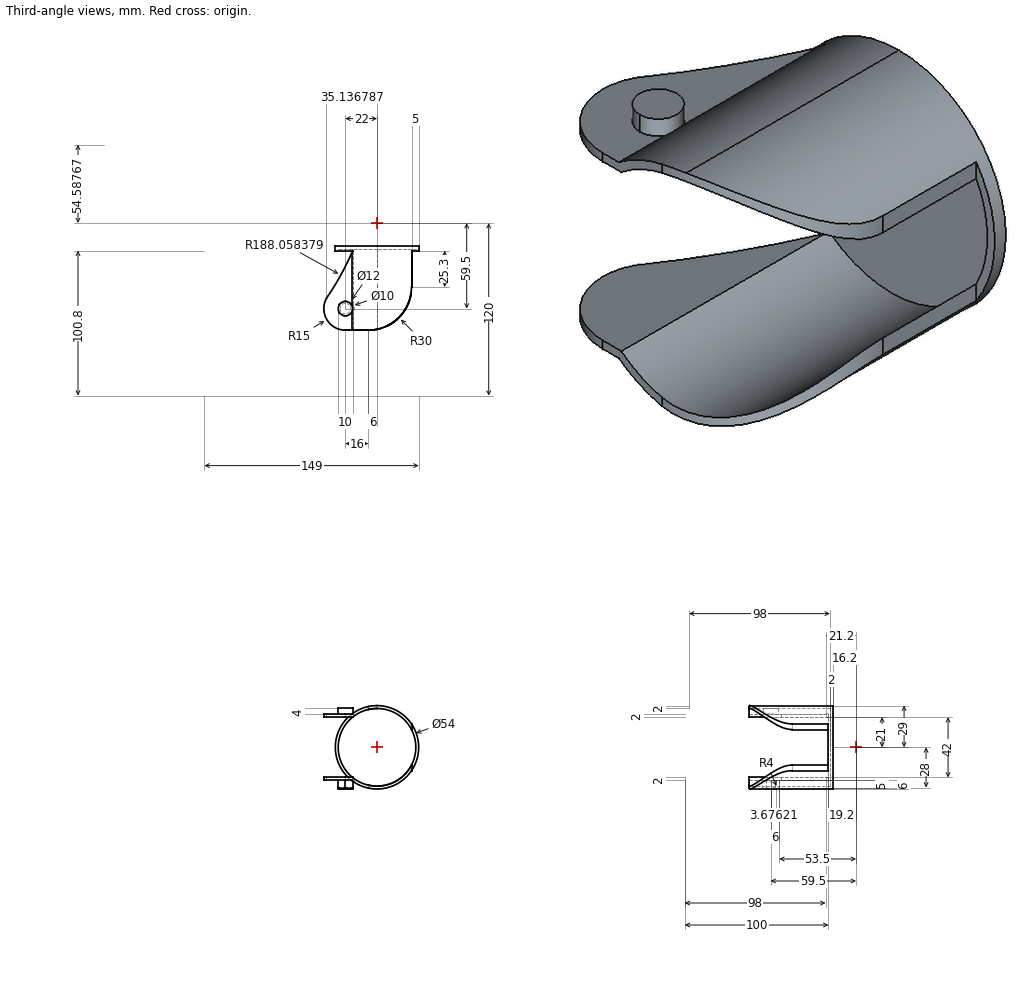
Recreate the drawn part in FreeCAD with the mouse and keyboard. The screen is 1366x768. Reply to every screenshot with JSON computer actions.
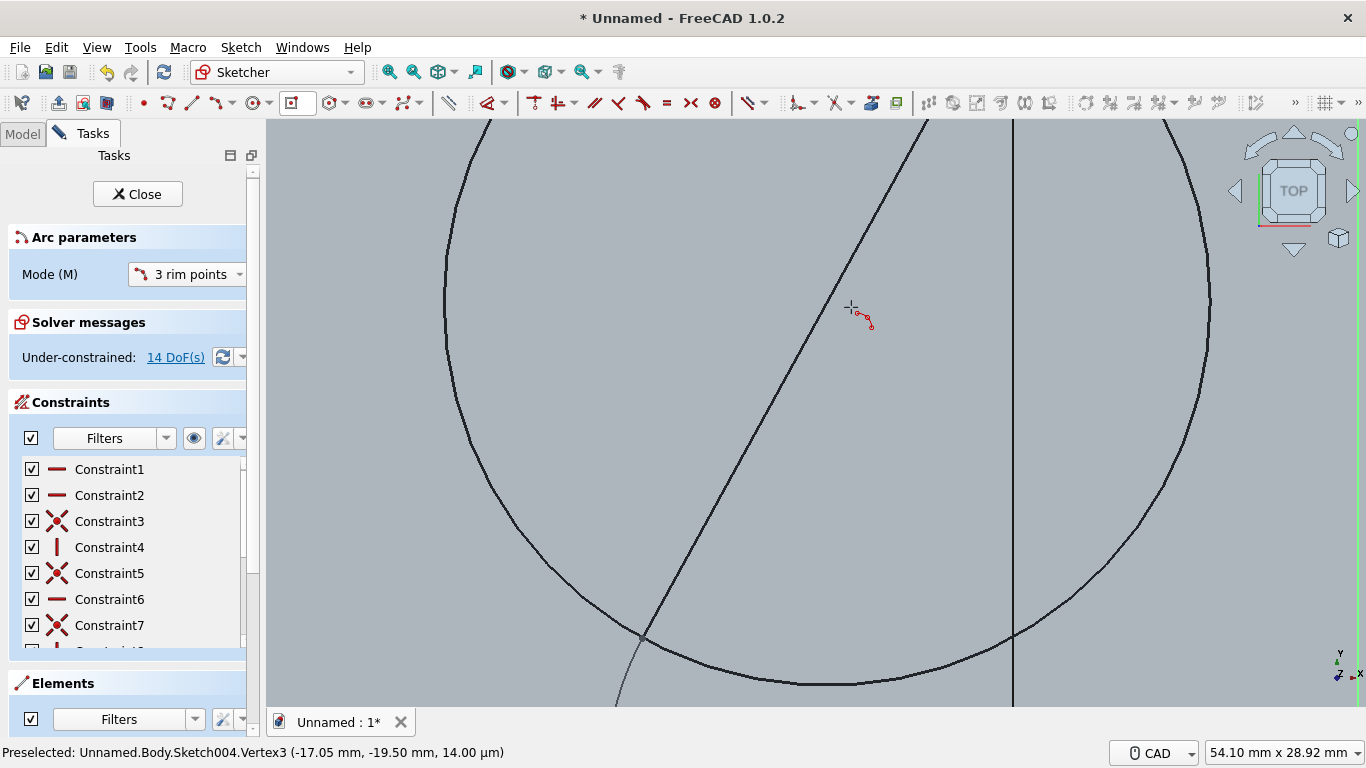
{"action": "left_click", "coordinate": [846, 306]}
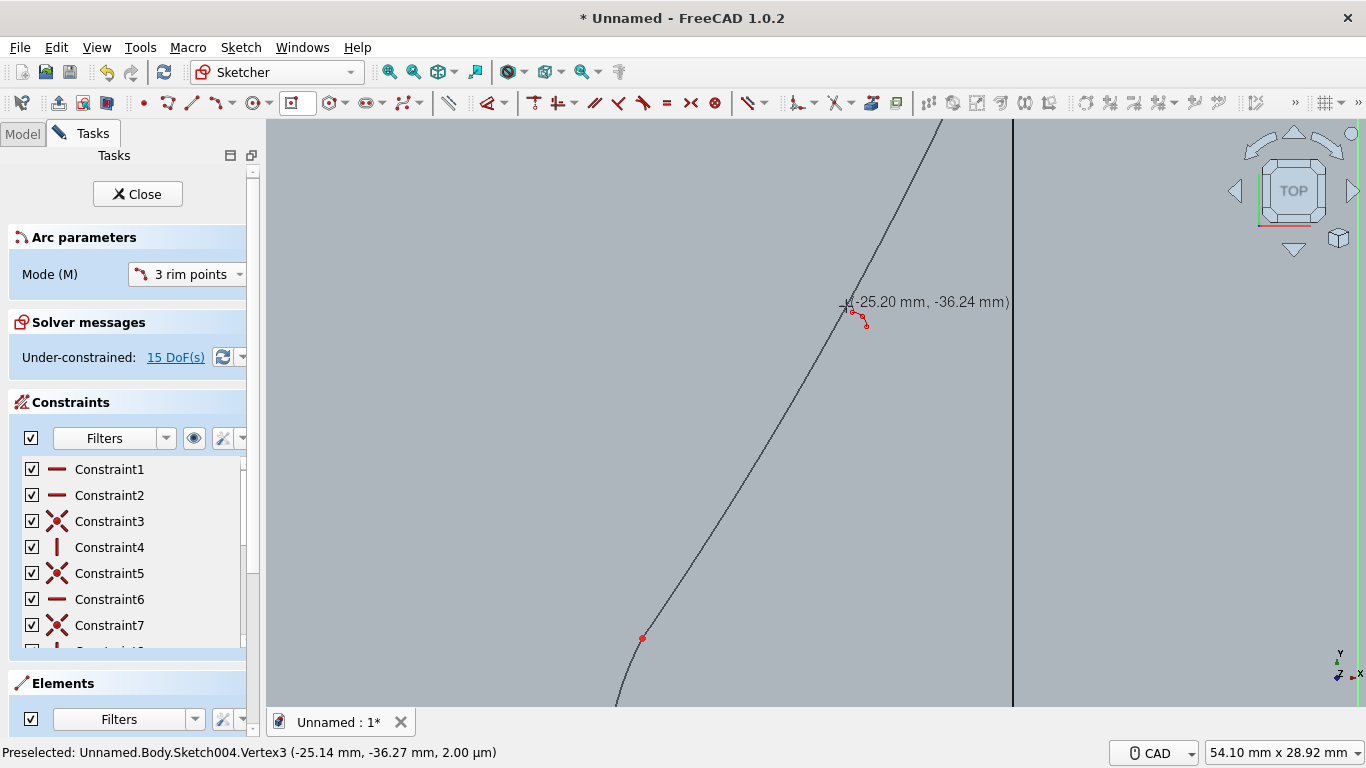
{"action": "scroll", "coordinate": [810, 338], "scroll_direction": "down", "scroll_amount": 9}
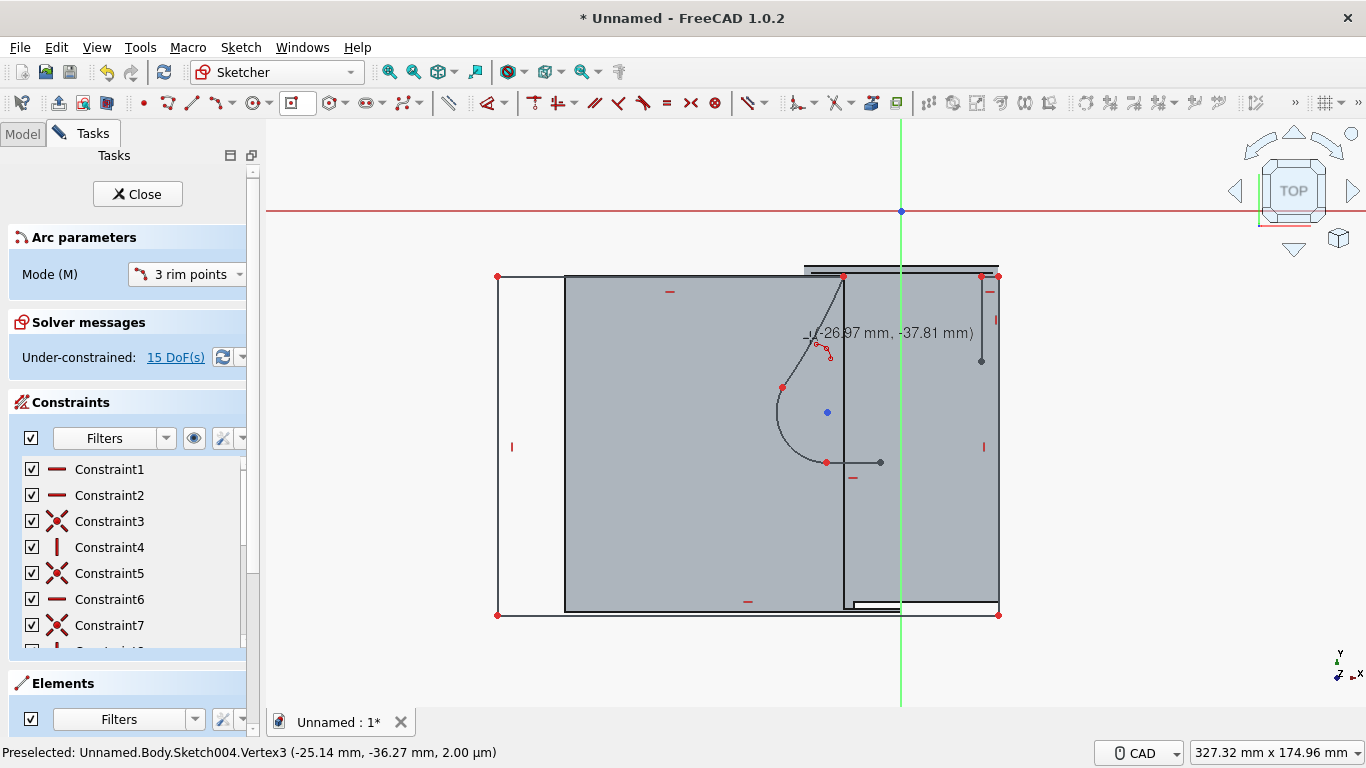
{"action": "left_click", "coordinate": [982, 362]}
{"action": "left_click", "coordinate": [881, 463]}
{"action": "left_click", "coordinate": [952, 432]}
{"action": "key", "text": "Escape"}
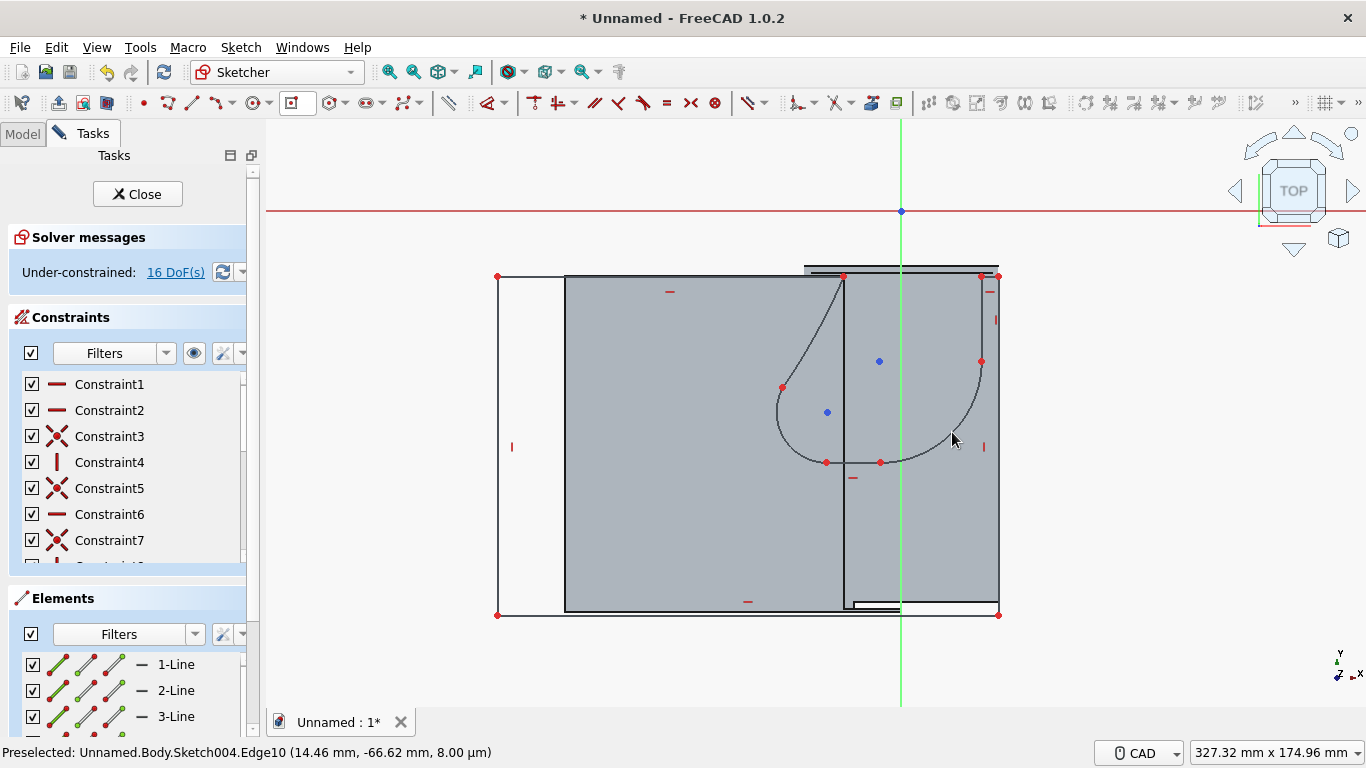
{"action": "left_click", "coordinate": [865, 463]}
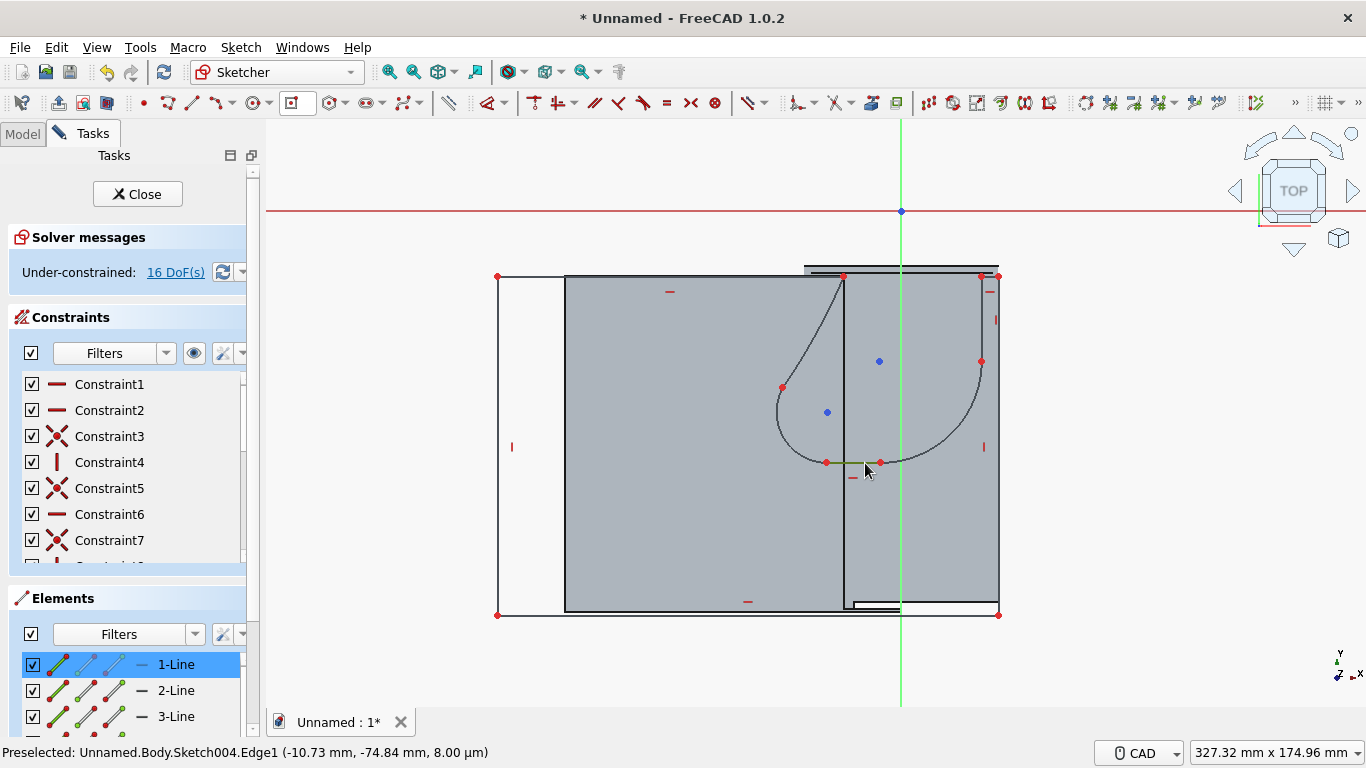
{"action": "left_click", "coordinate": [777, 418]}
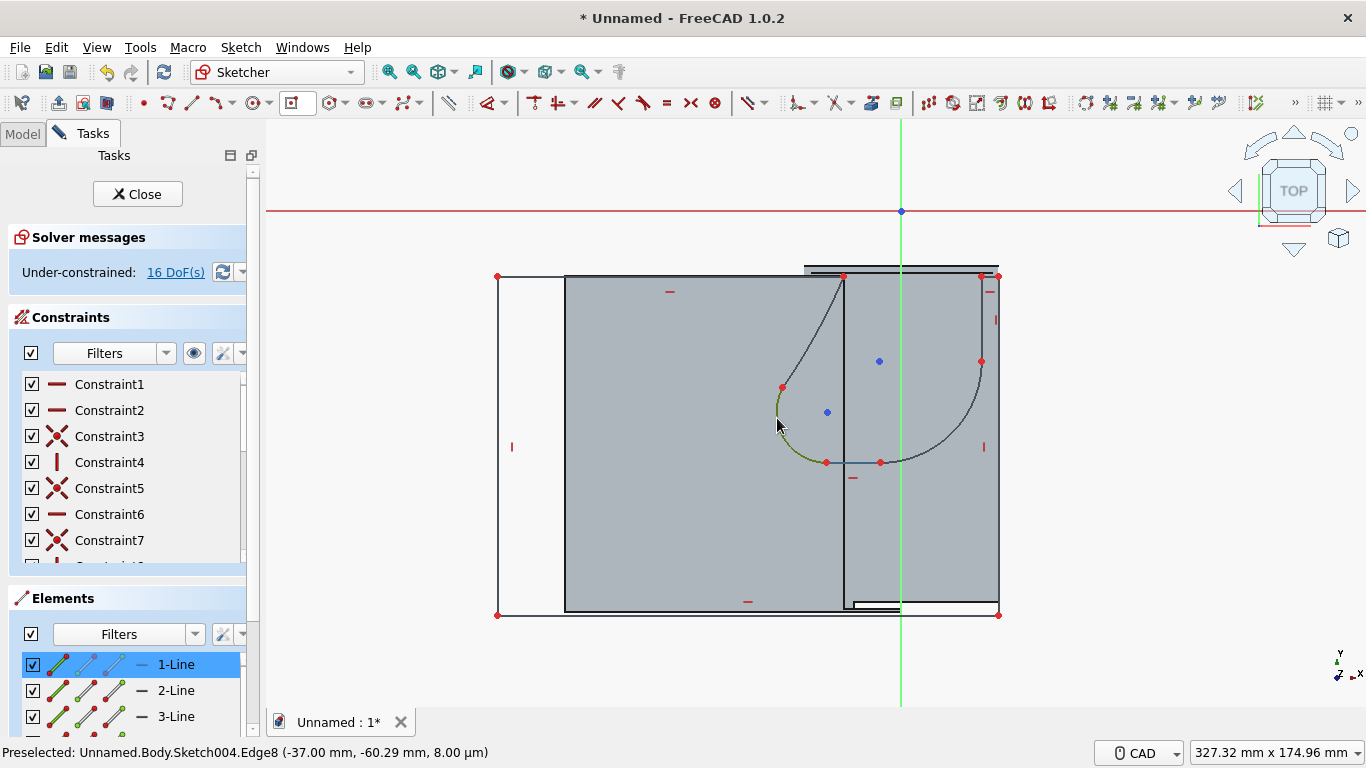
{"action": "left_click", "coordinate": [644, 104]}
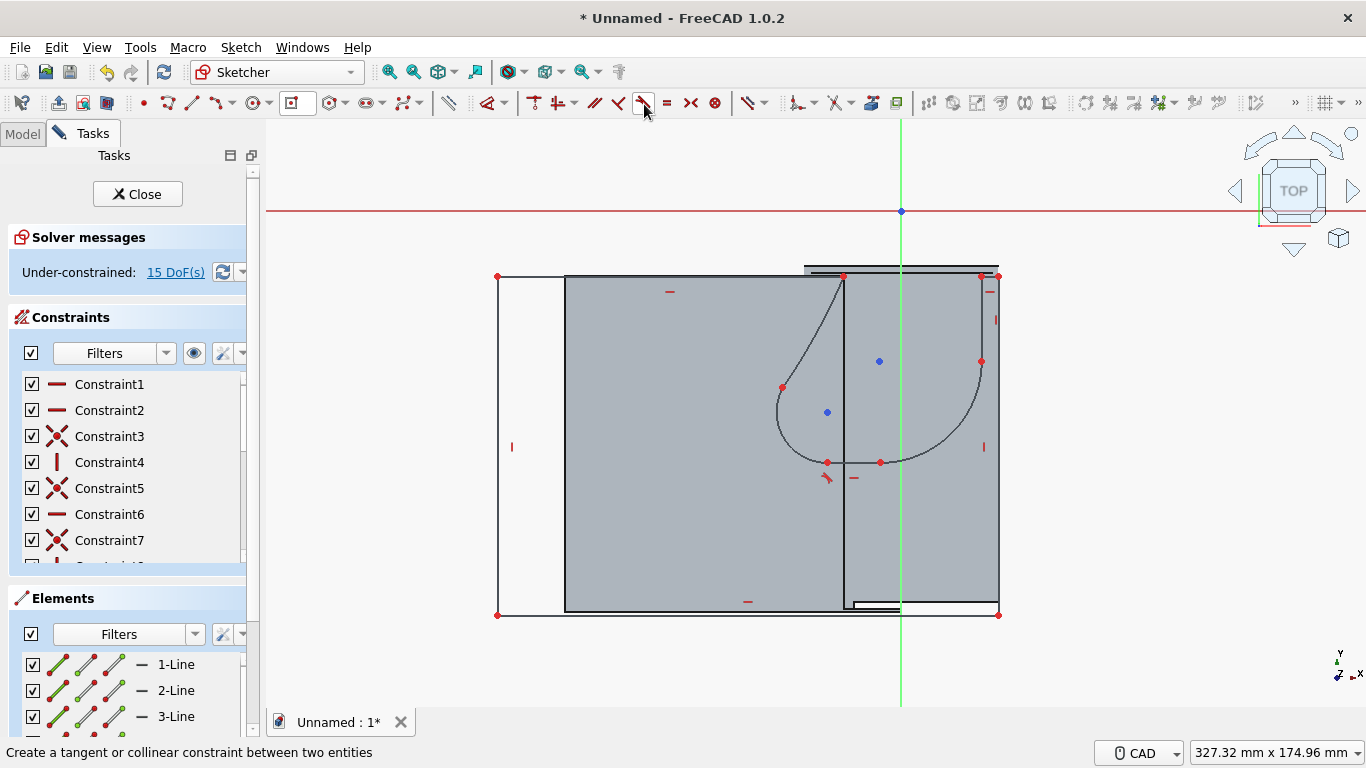
{"action": "left_click", "coordinate": [865, 463]}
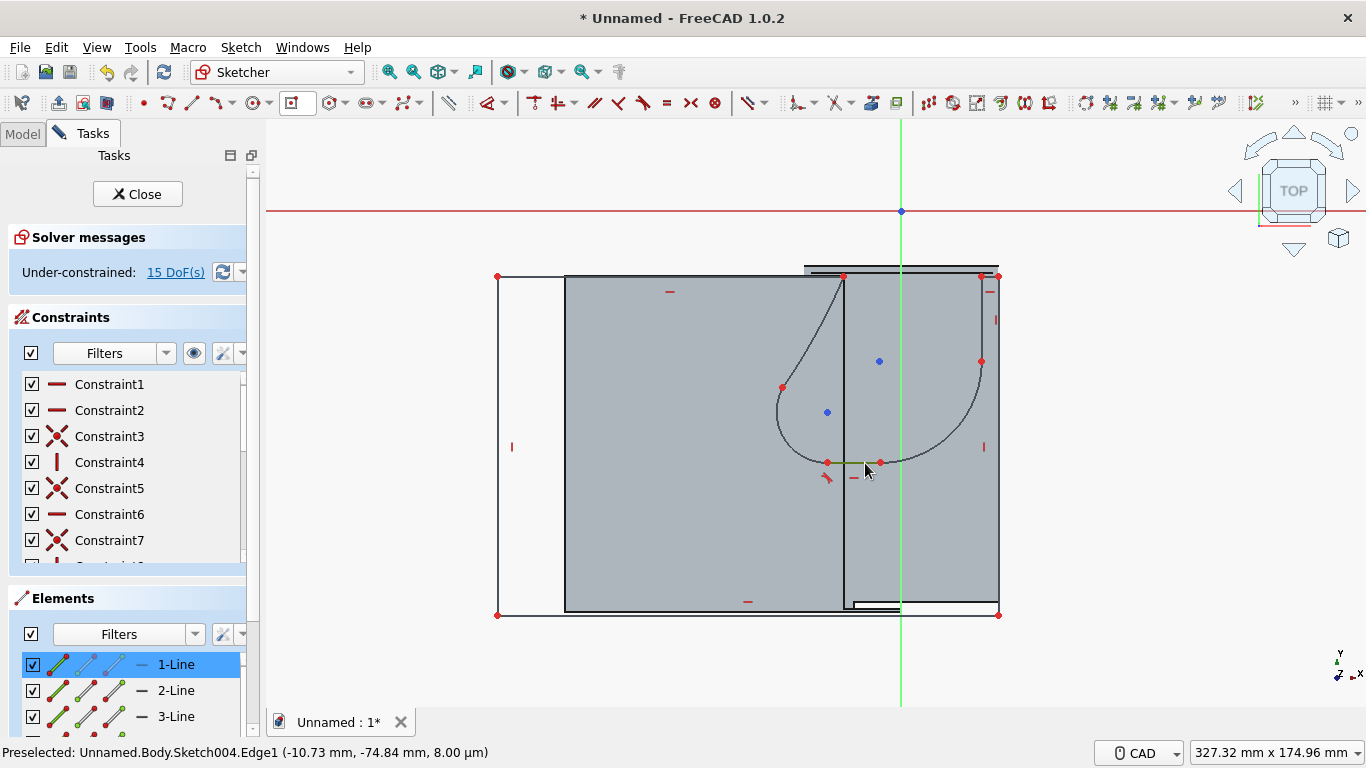
{"action": "left_click", "coordinate": [926, 452]}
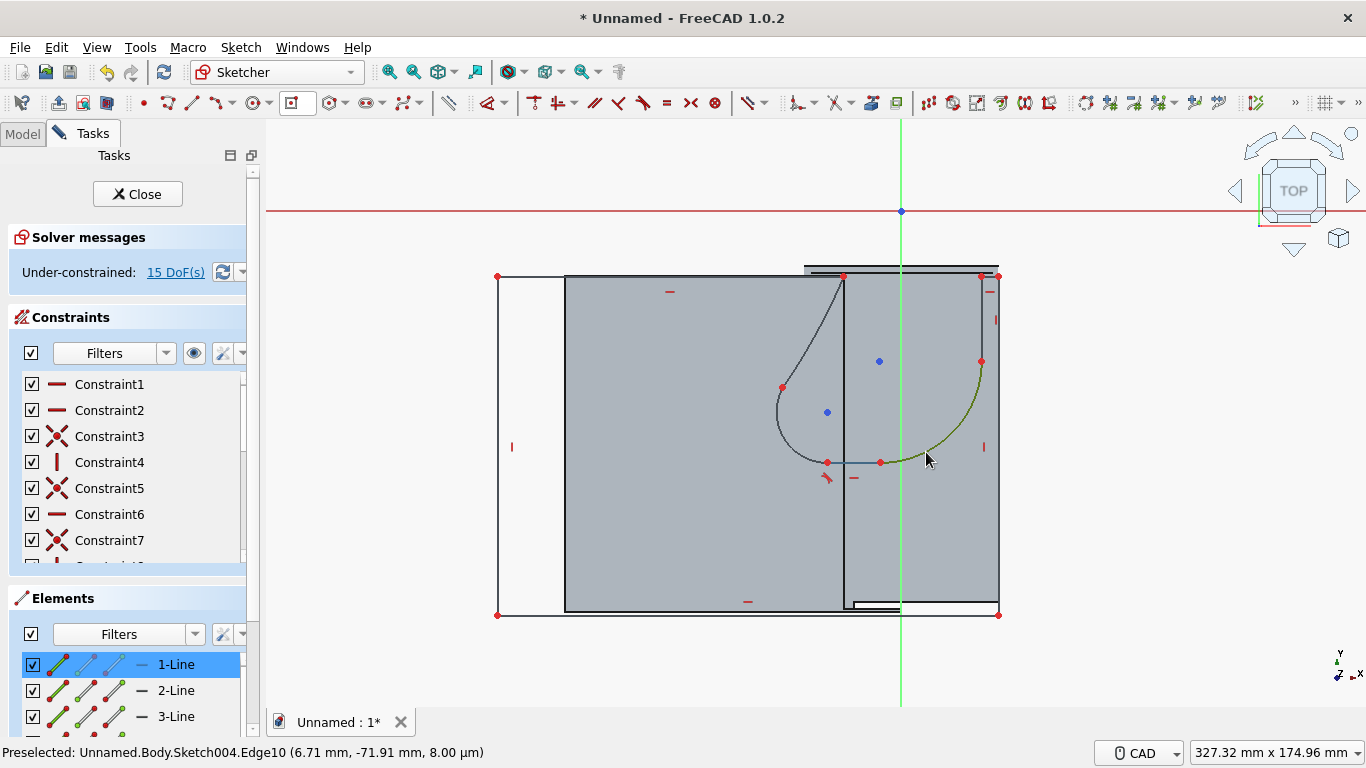
{"action": "left_click", "coordinate": [644, 104]}